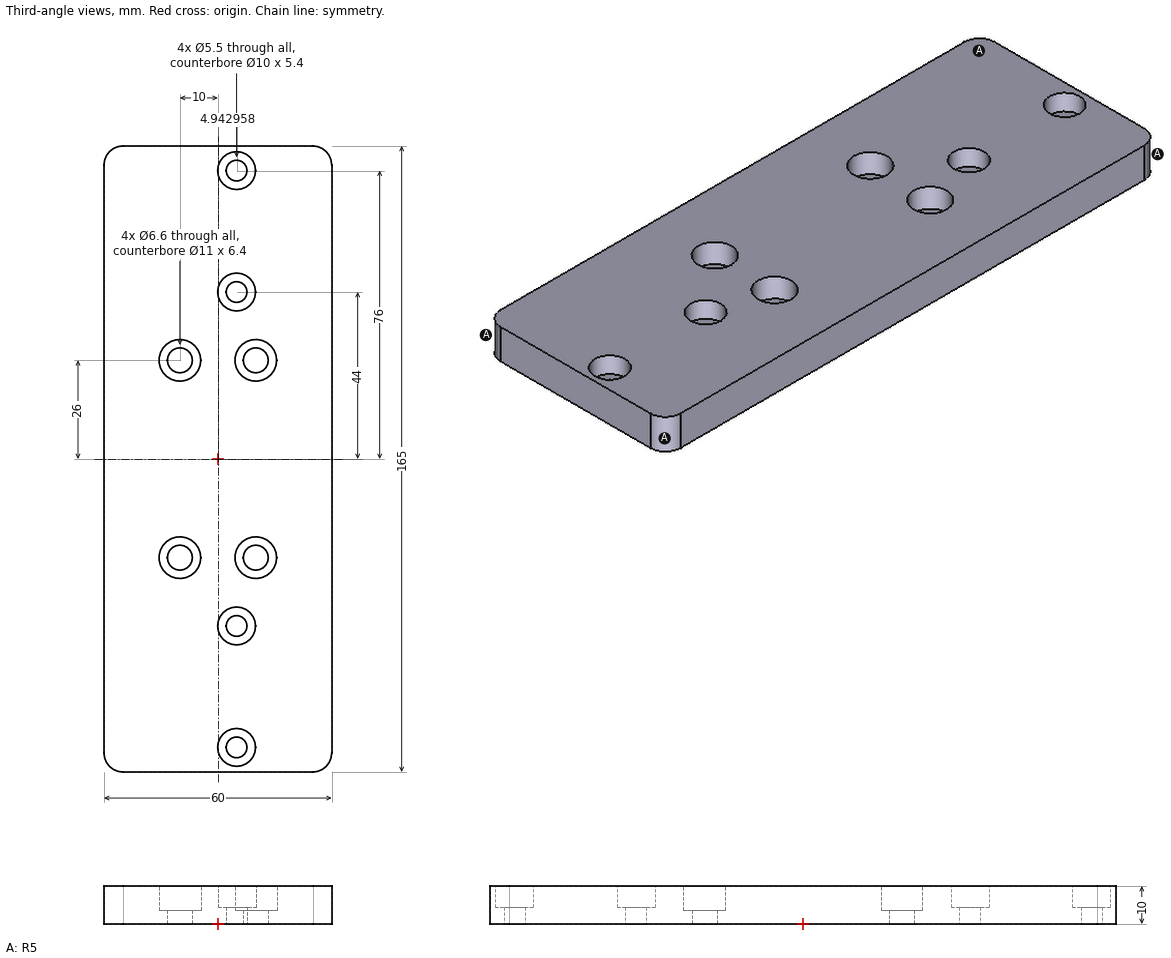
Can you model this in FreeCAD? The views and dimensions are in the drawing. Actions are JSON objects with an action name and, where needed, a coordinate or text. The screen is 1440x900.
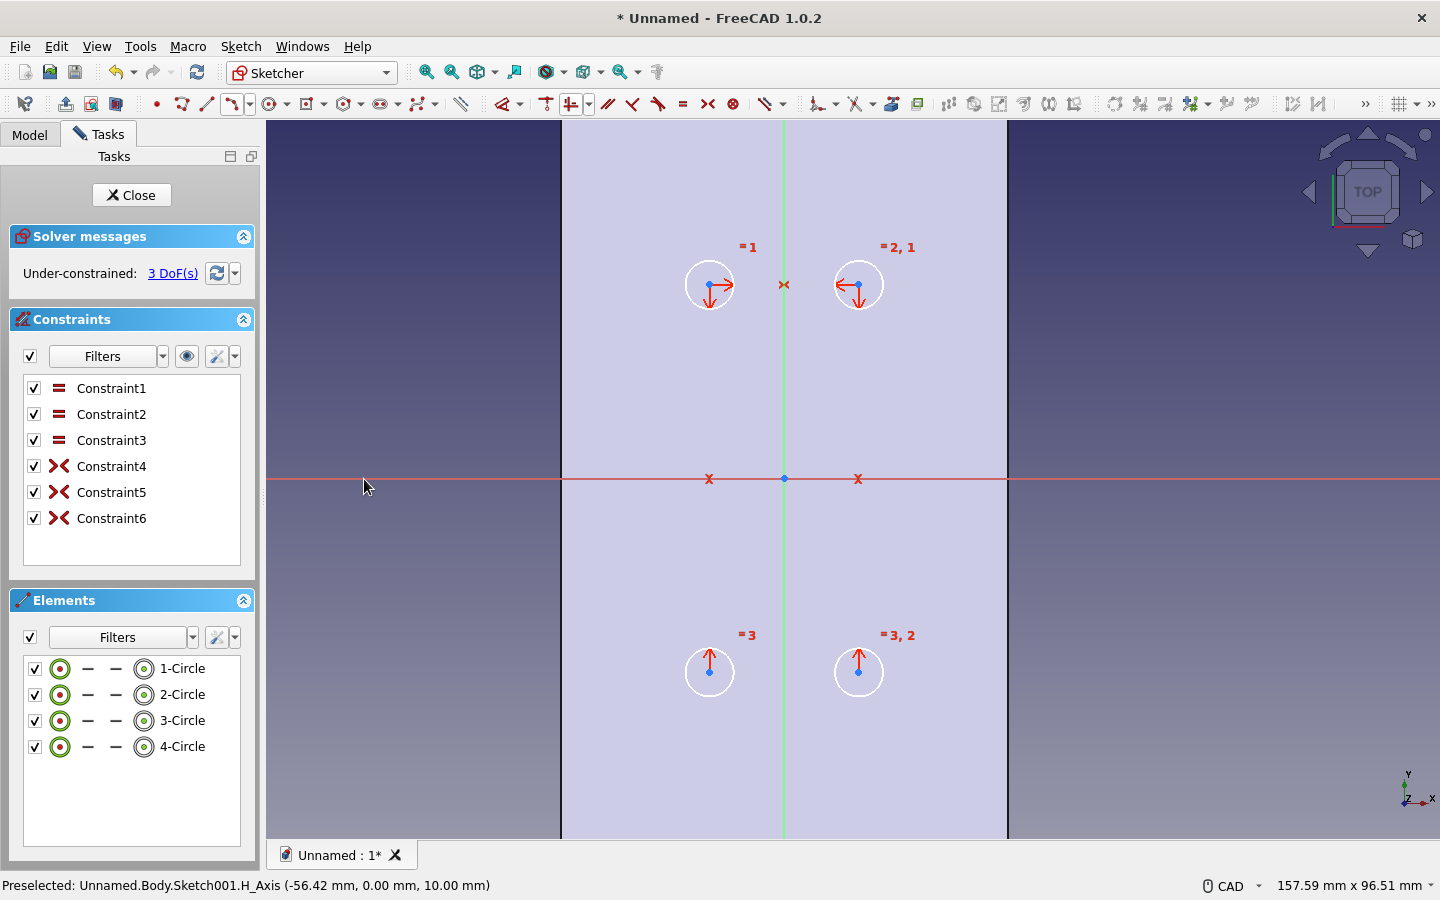
{"action": "left_click", "coordinate": [502, 104]}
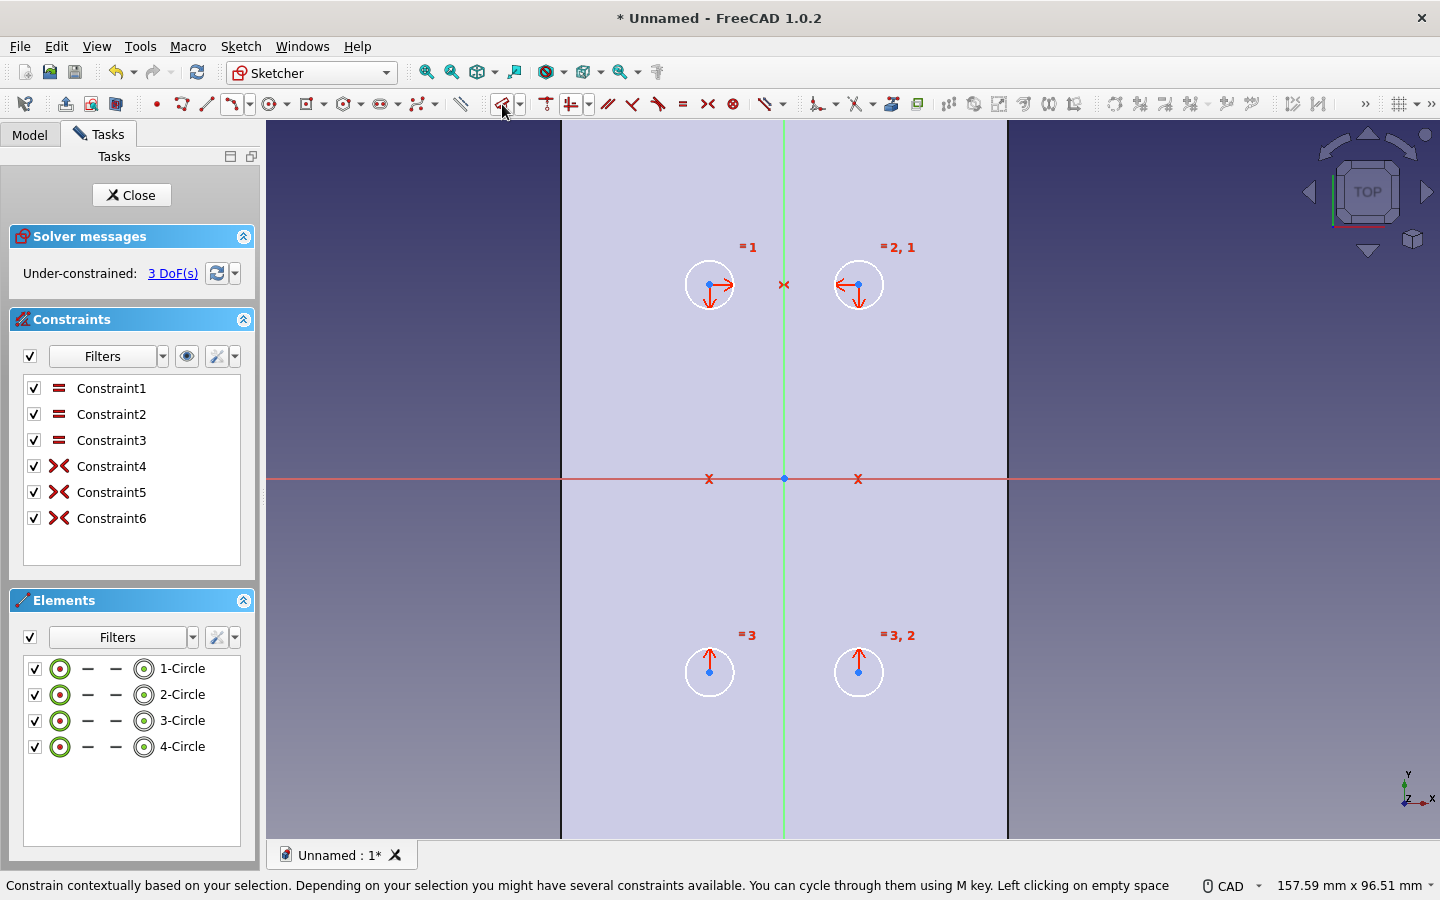
{"action": "left_click", "coordinate": [727, 268]}
{"action": "left_click", "coordinate": [750, 246]}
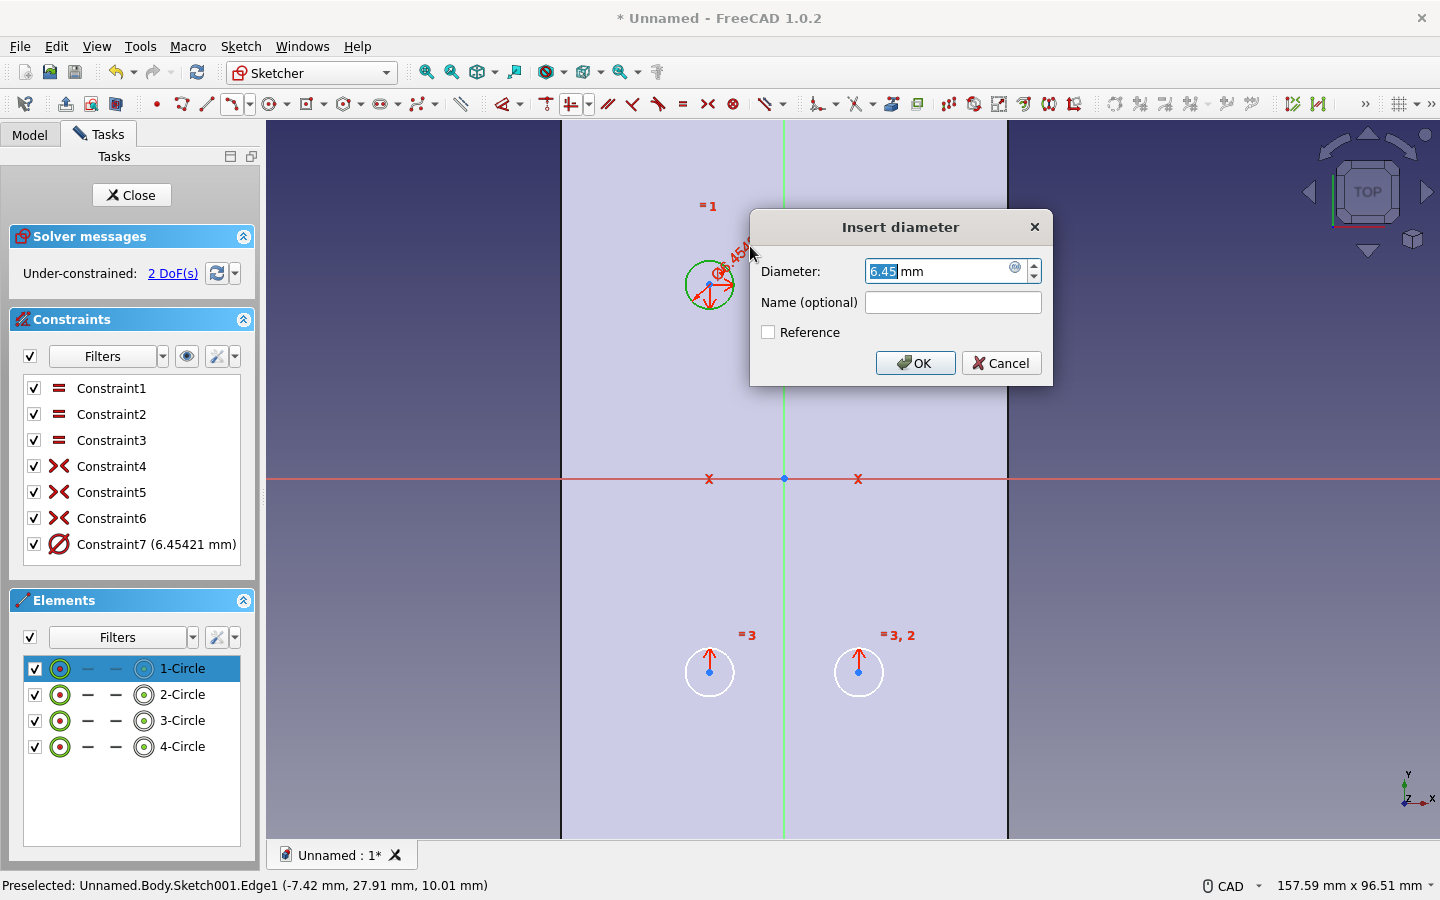
{"action": "type", "text": "6.6"}
{"action": "key", "text": "Return"}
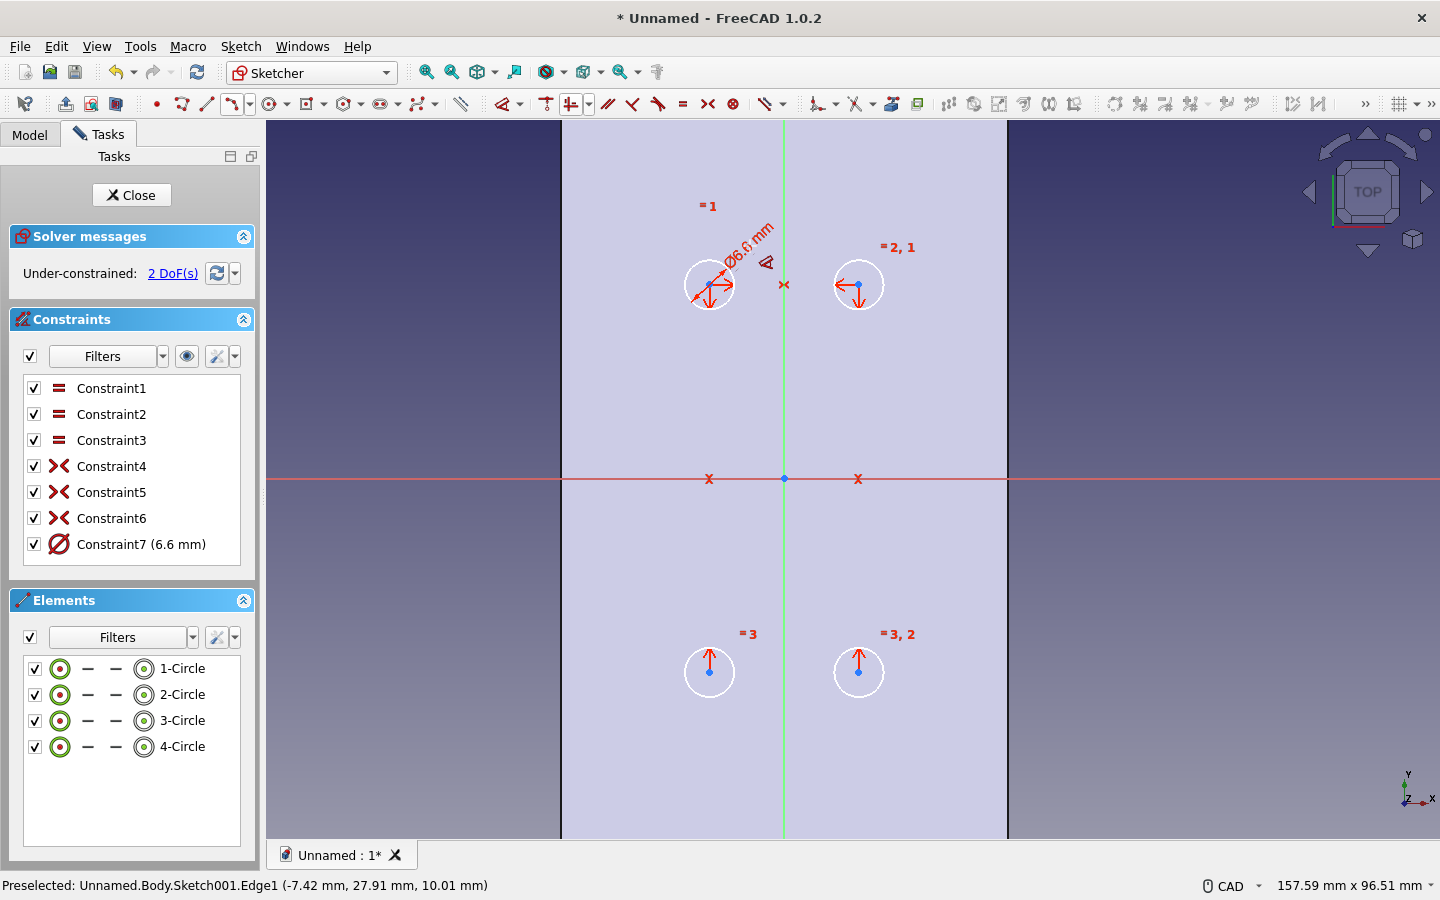
{"action": "left_click", "coordinate": [710, 285]}
{"action": "left_click", "coordinate": [747, 513]}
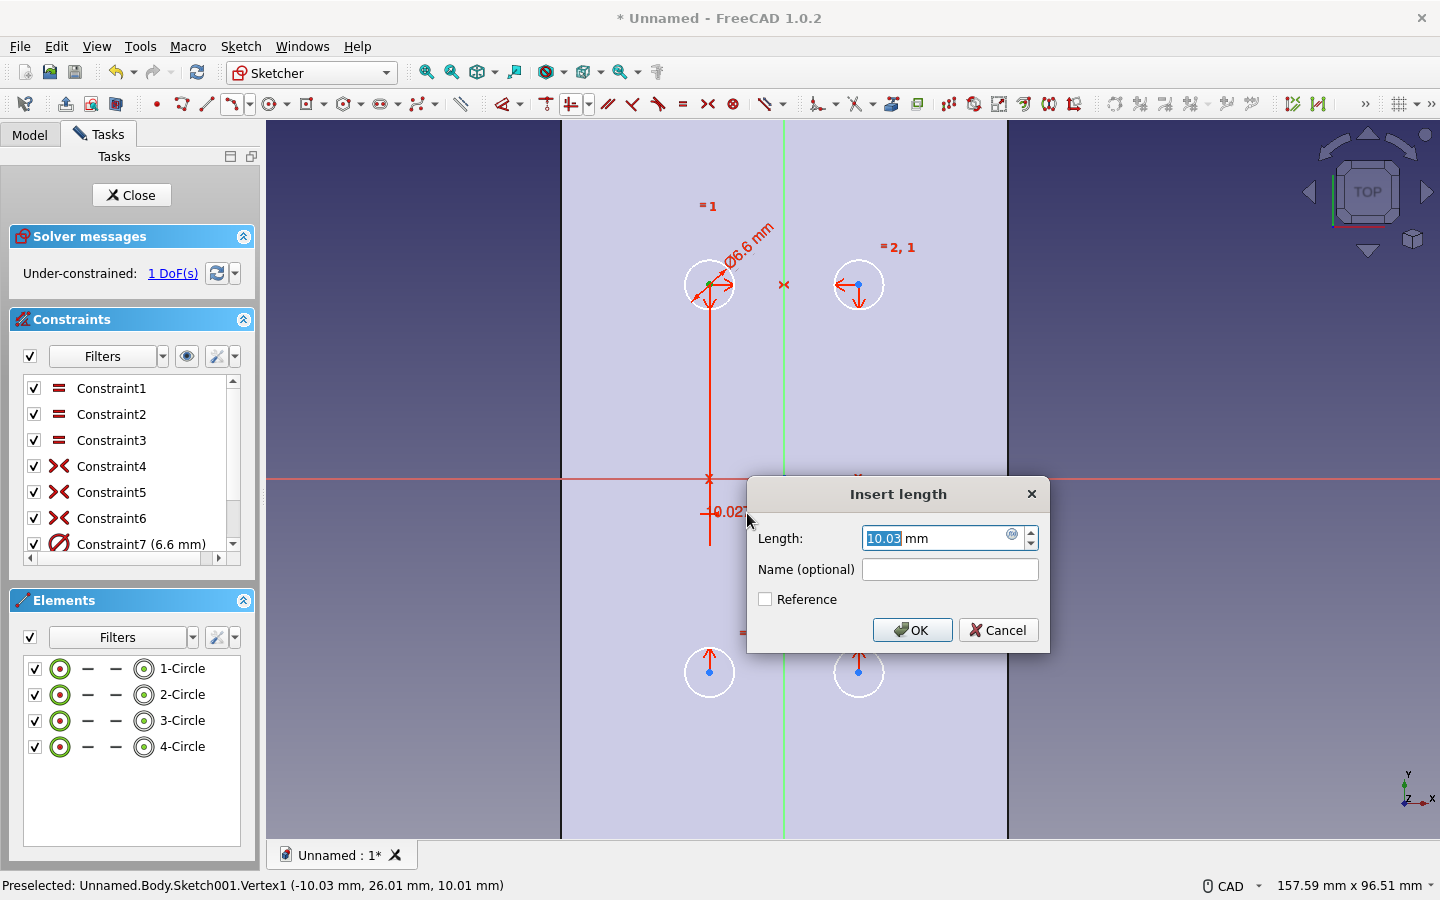
{"action": "type", "text": "10"}
{"action": "key", "text": "Return"}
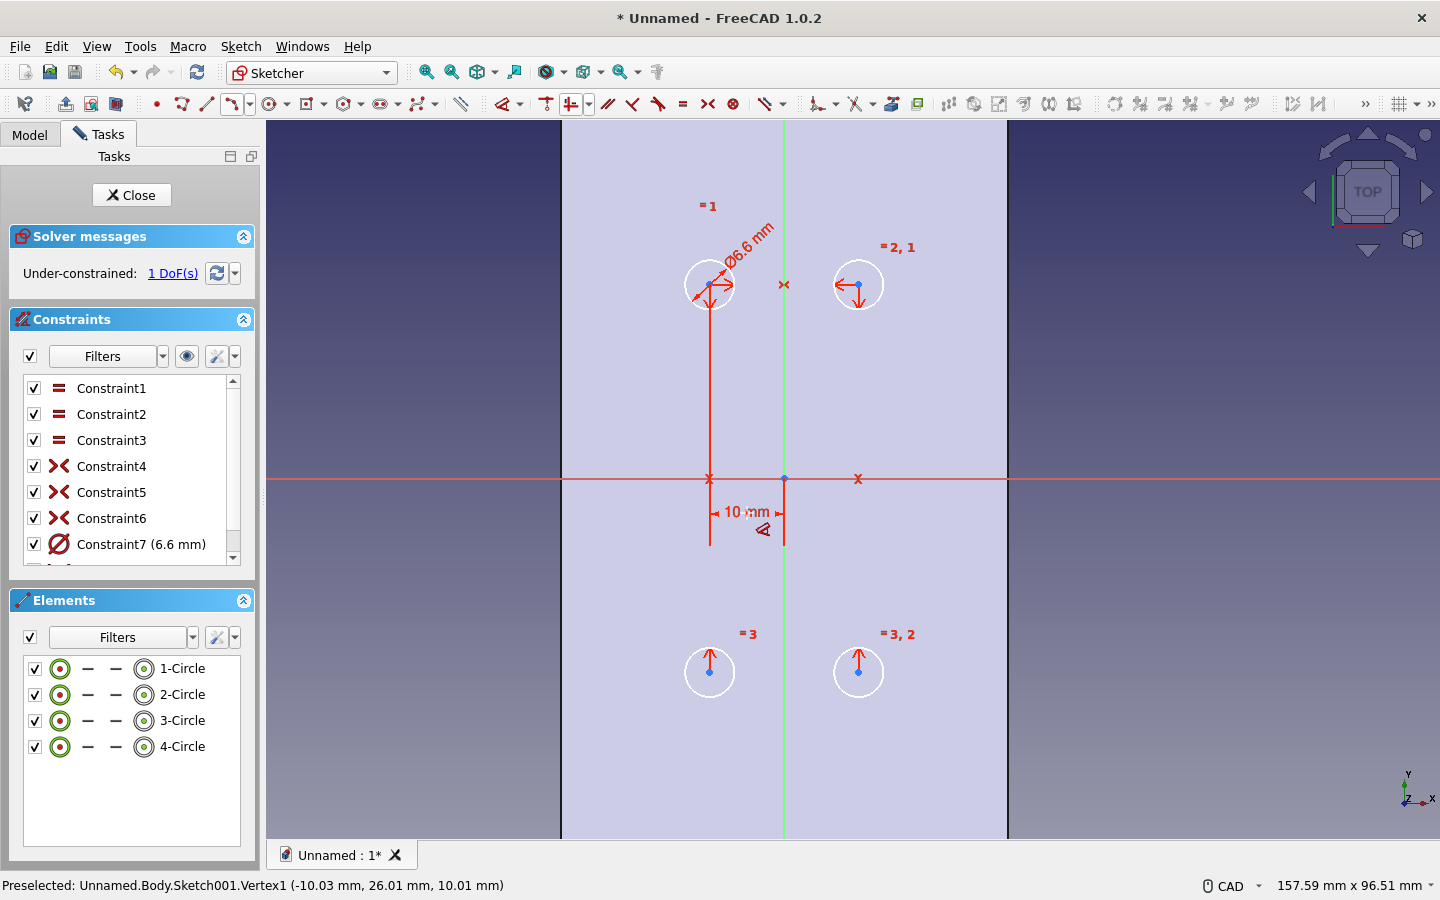
{"action": "left_click", "coordinate": [710, 285]}
{"action": "left_click", "coordinate": [676, 382]}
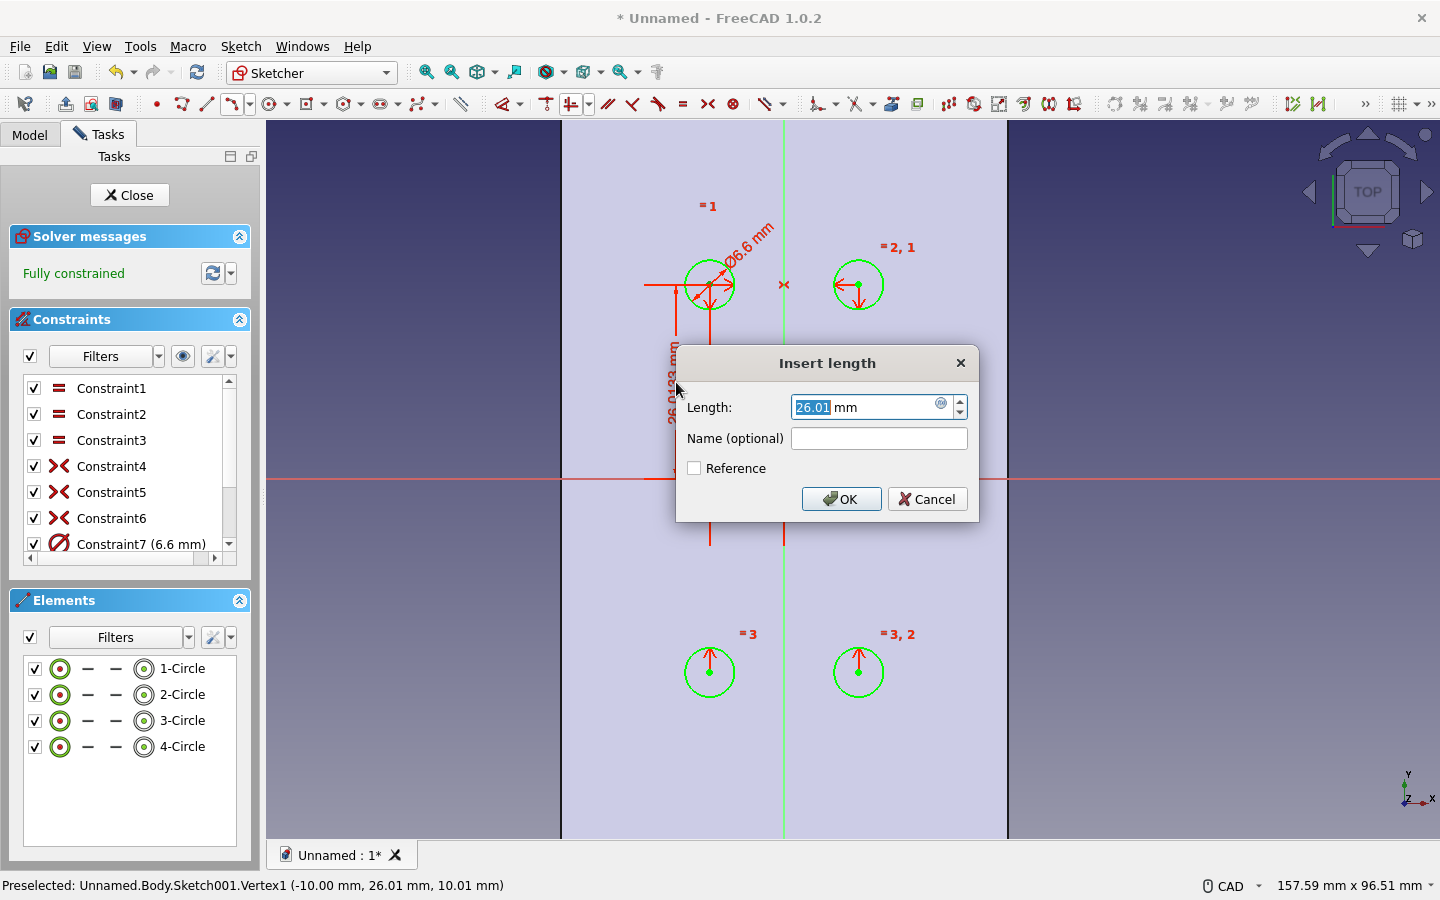
{"action": "type", "text": "26"}
{"action": "key", "text": "Return"}
{"action": "key", "text": "Escape"}